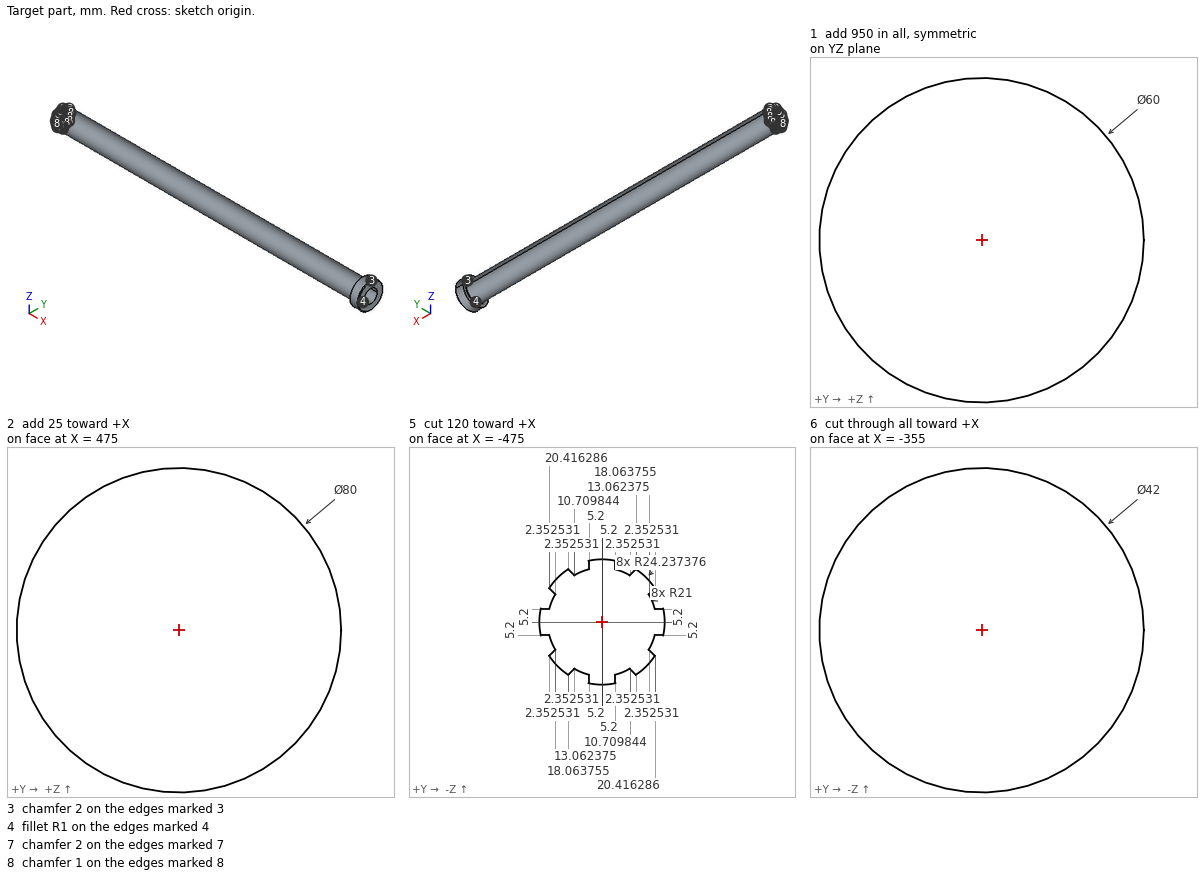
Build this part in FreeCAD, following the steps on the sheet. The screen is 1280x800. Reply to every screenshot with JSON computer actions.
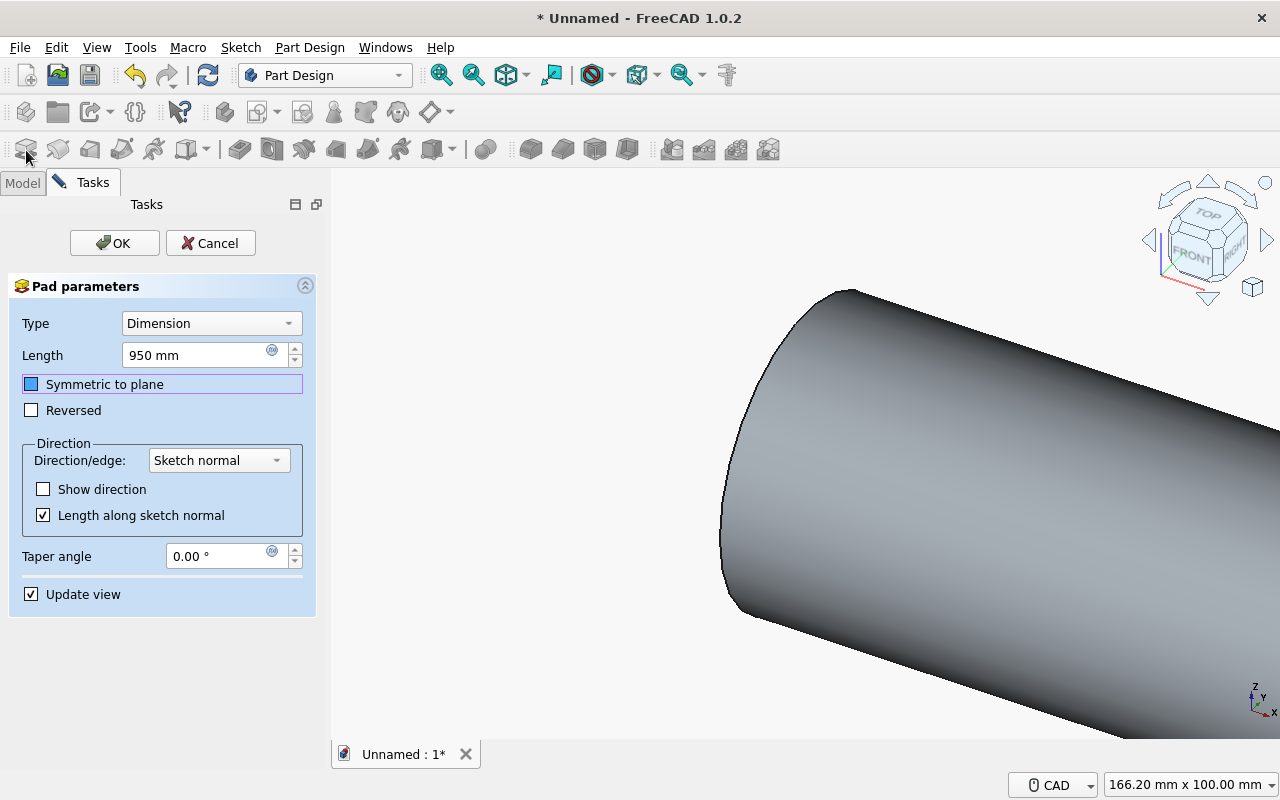
{"action": "left_click", "coordinate": [30, 384]}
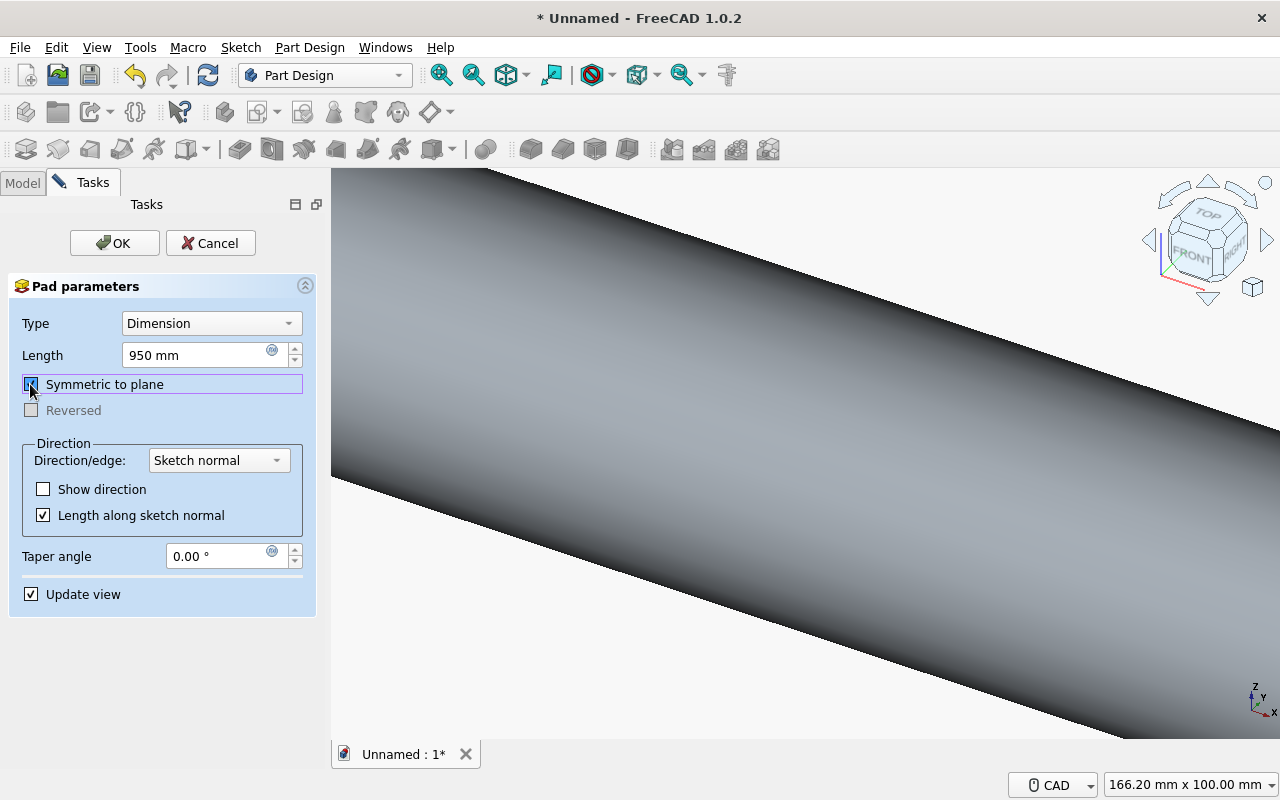
{"action": "left_click", "coordinate": [115, 243]}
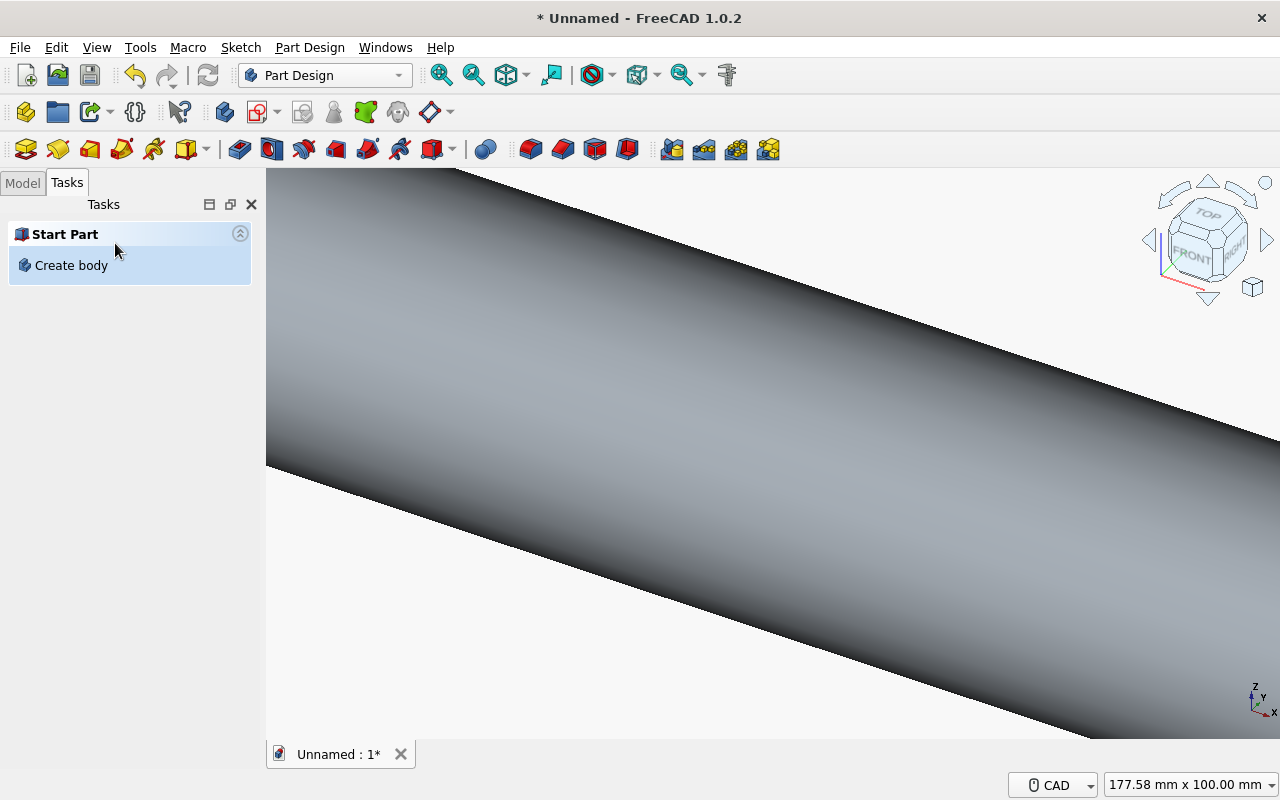
{"action": "left_click", "coordinate": [442, 76]}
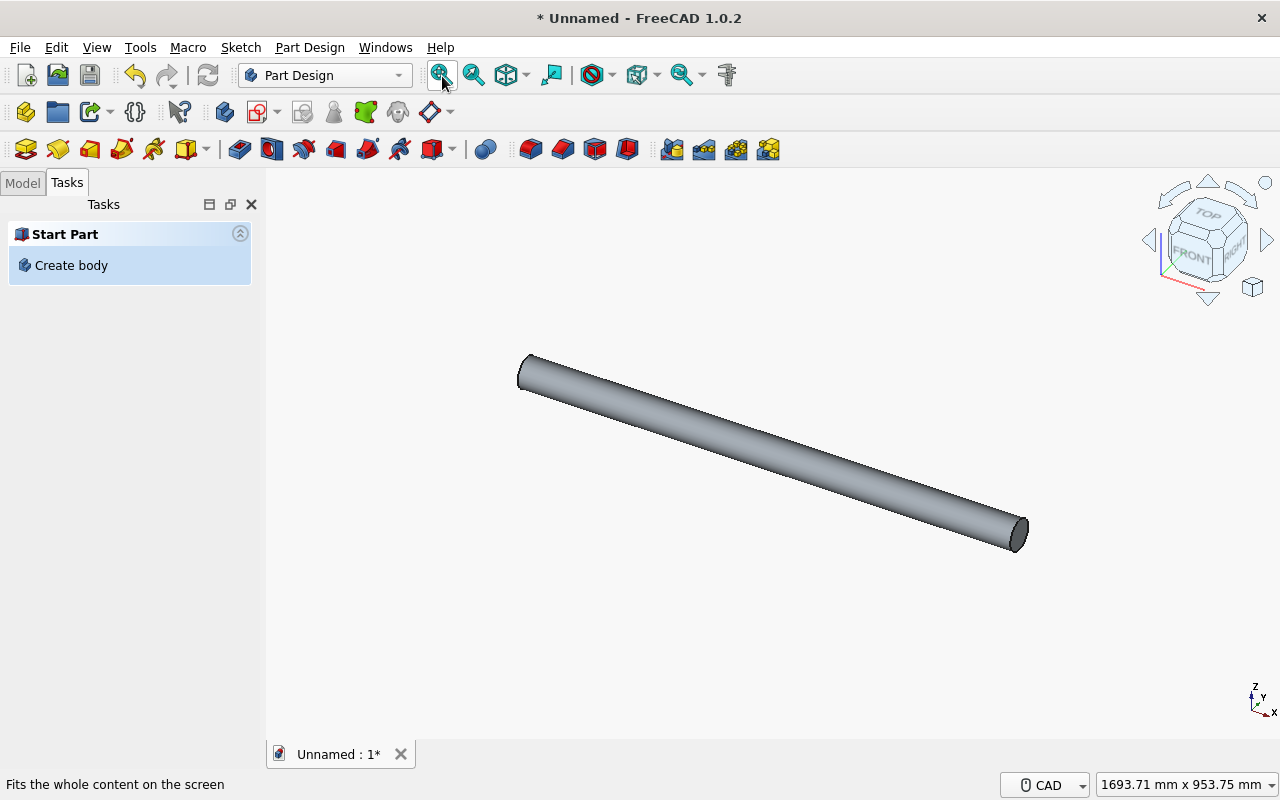
{"action": "left_click", "coordinate": [1022, 532]}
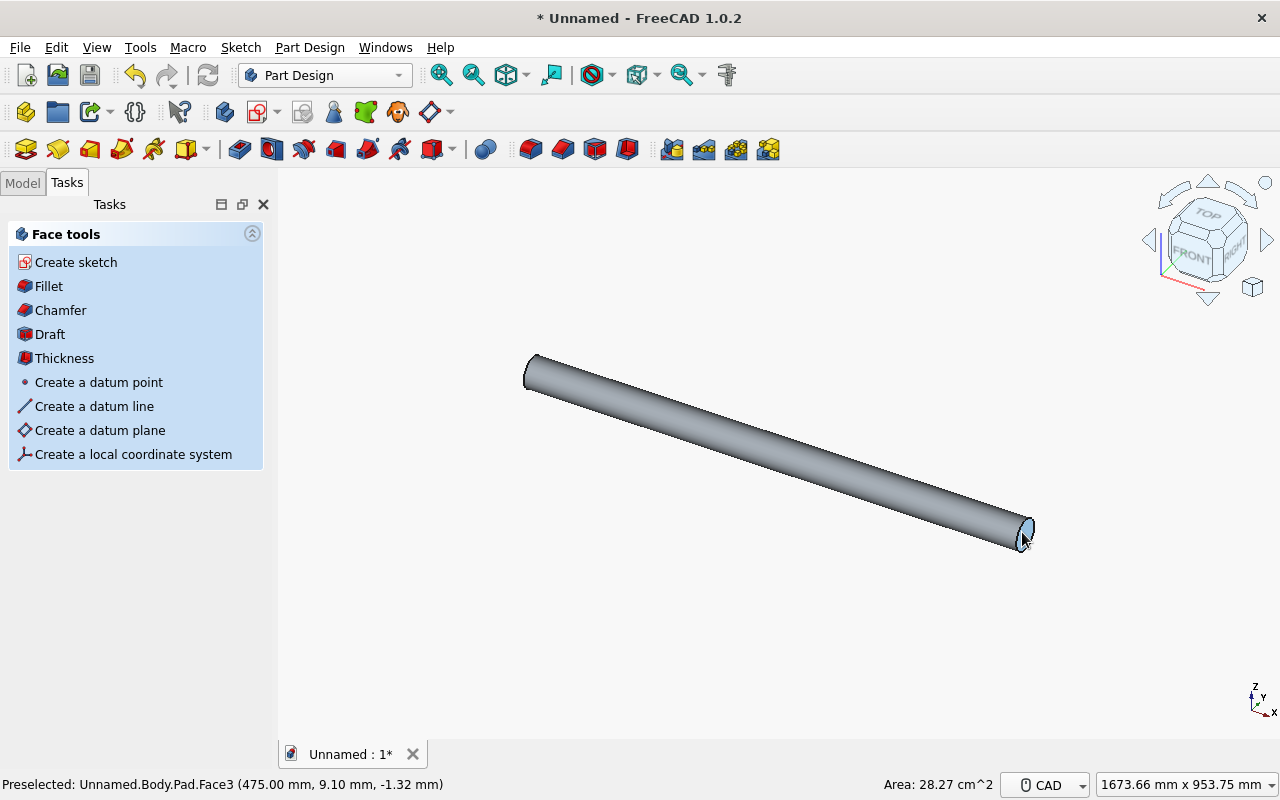
{"action": "left_click", "coordinate": [258, 112]}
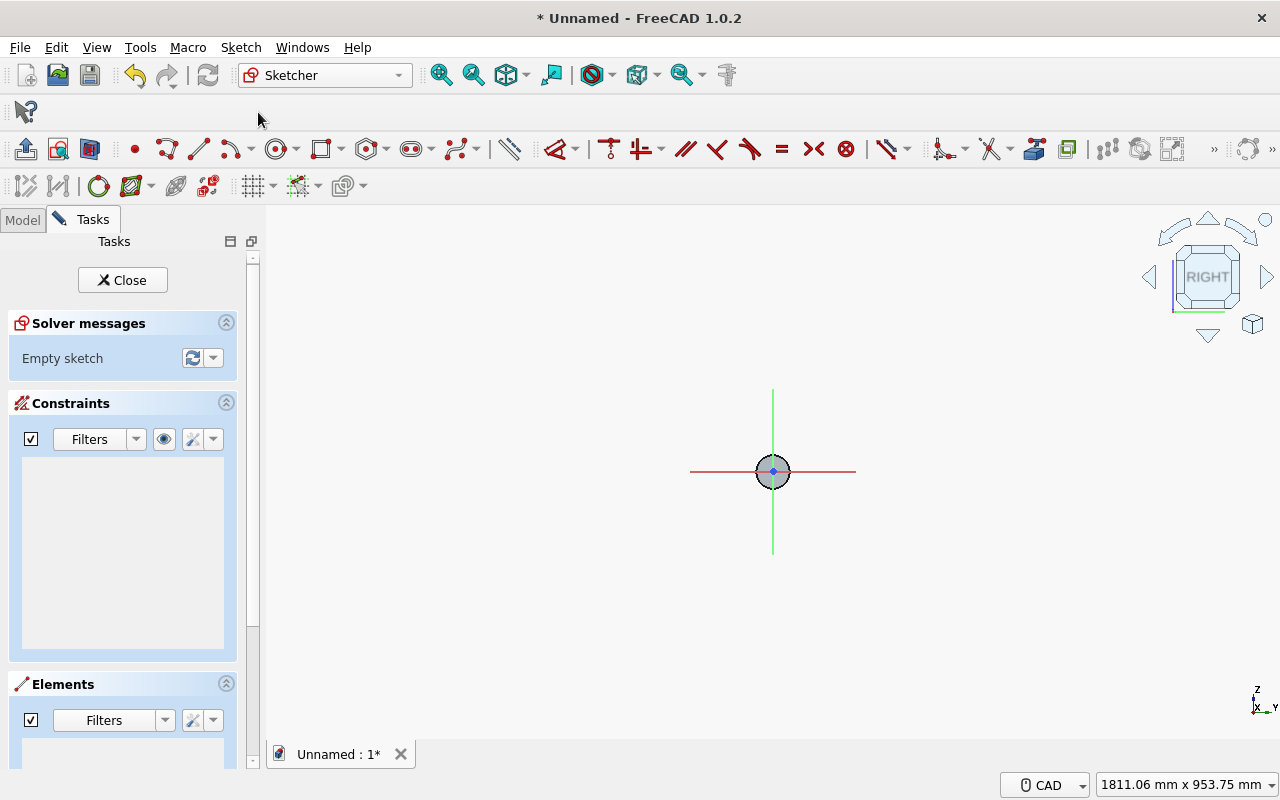
{"action": "scroll", "coordinate": [784, 472], "scroll_direction": "up", "scroll_amount": 10}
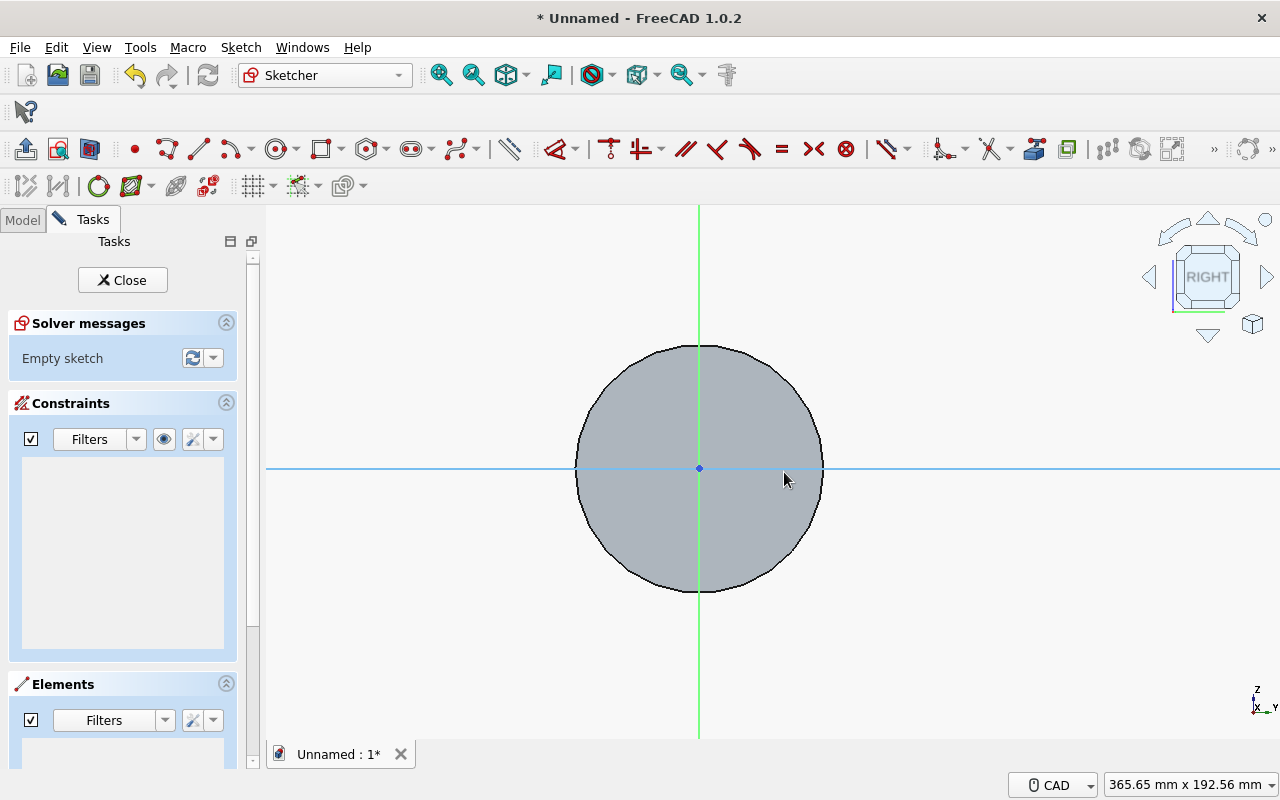
{"action": "key", "text": "g c"}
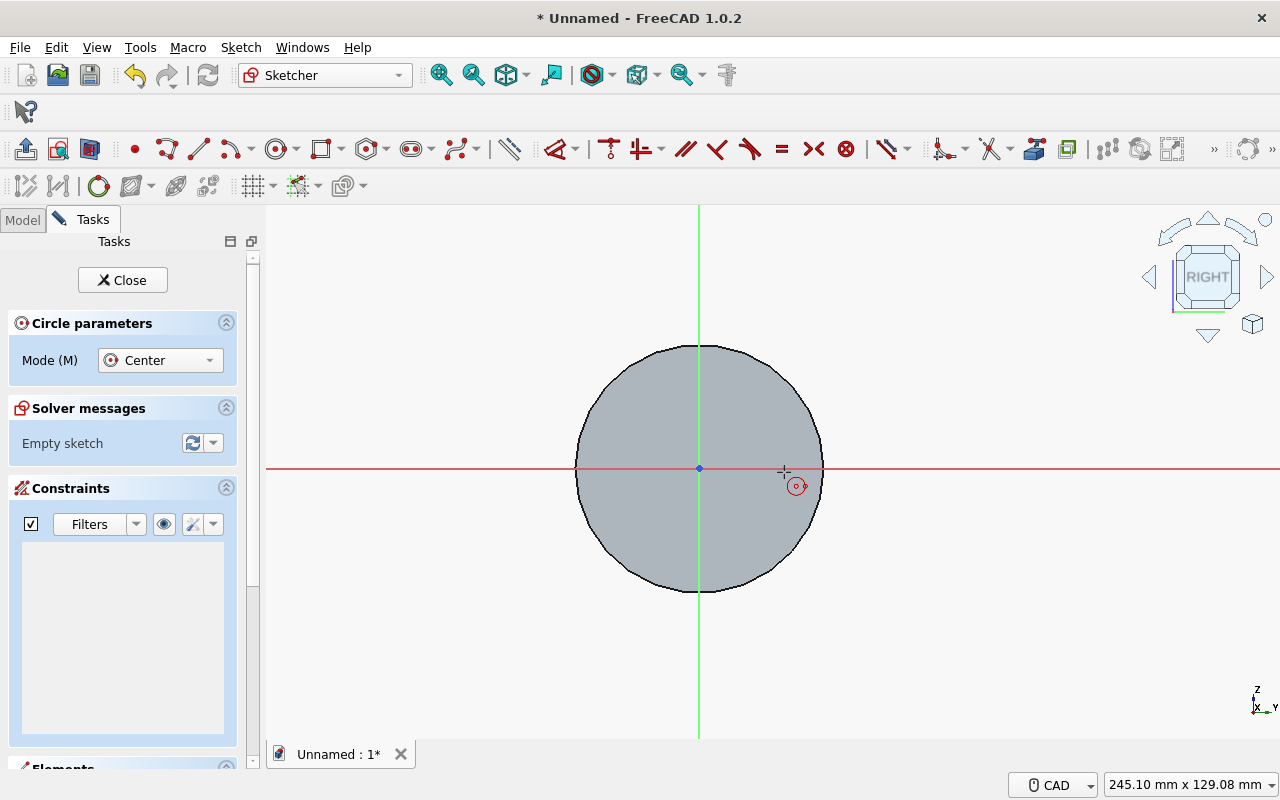
{"action": "left_click", "coordinate": [699, 469]}
{"action": "mouse_move", "coordinate": [816, 352]}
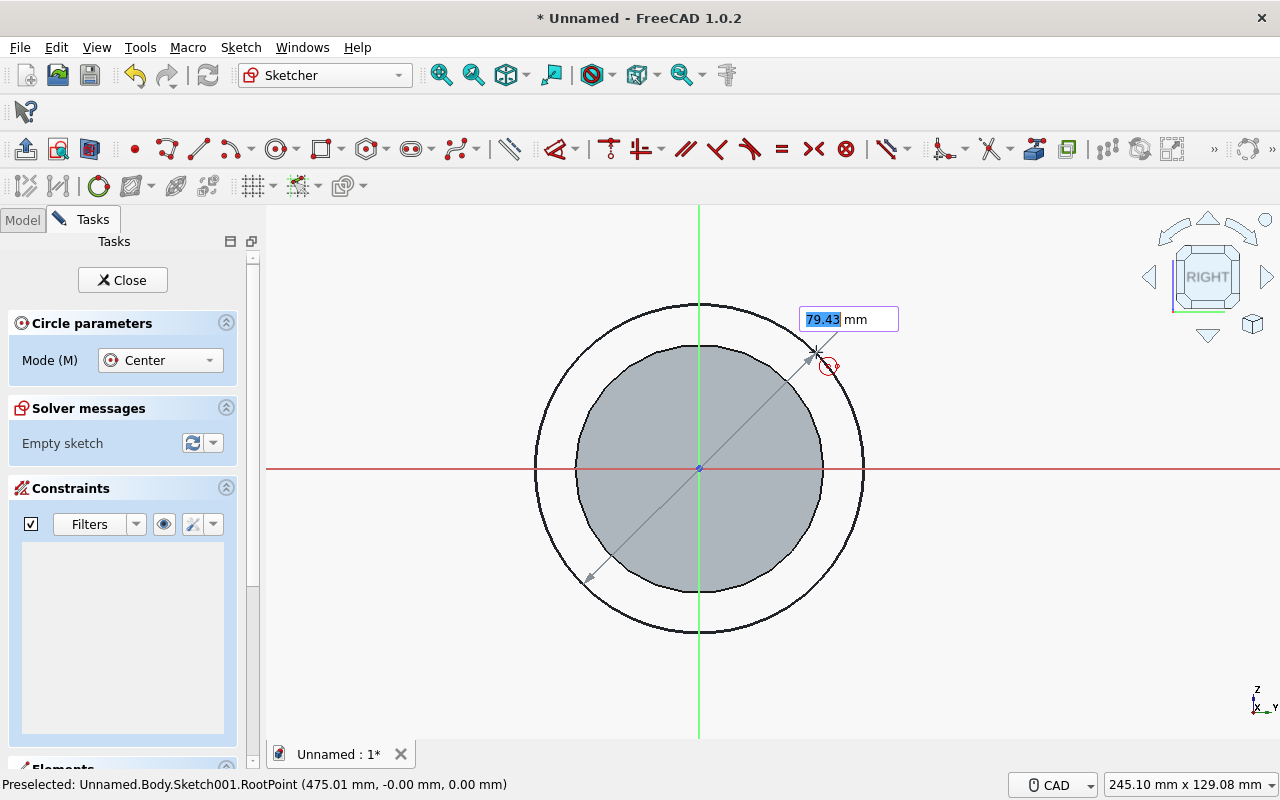
{"action": "type", "text": "80"}
{"action": "key", "text": "Return"}
{"action": "key", "text": "Escape"}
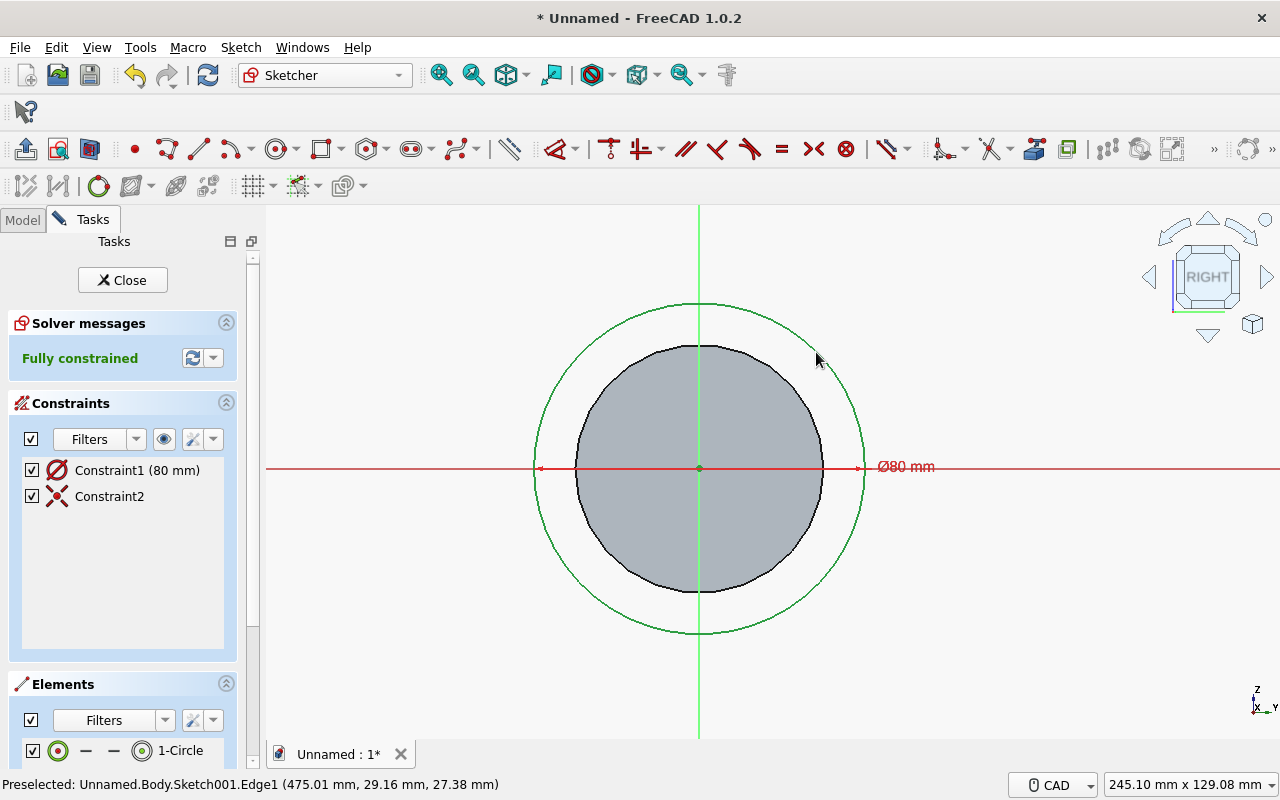
{"action": "left_click", "coordinate": [123, 280]}